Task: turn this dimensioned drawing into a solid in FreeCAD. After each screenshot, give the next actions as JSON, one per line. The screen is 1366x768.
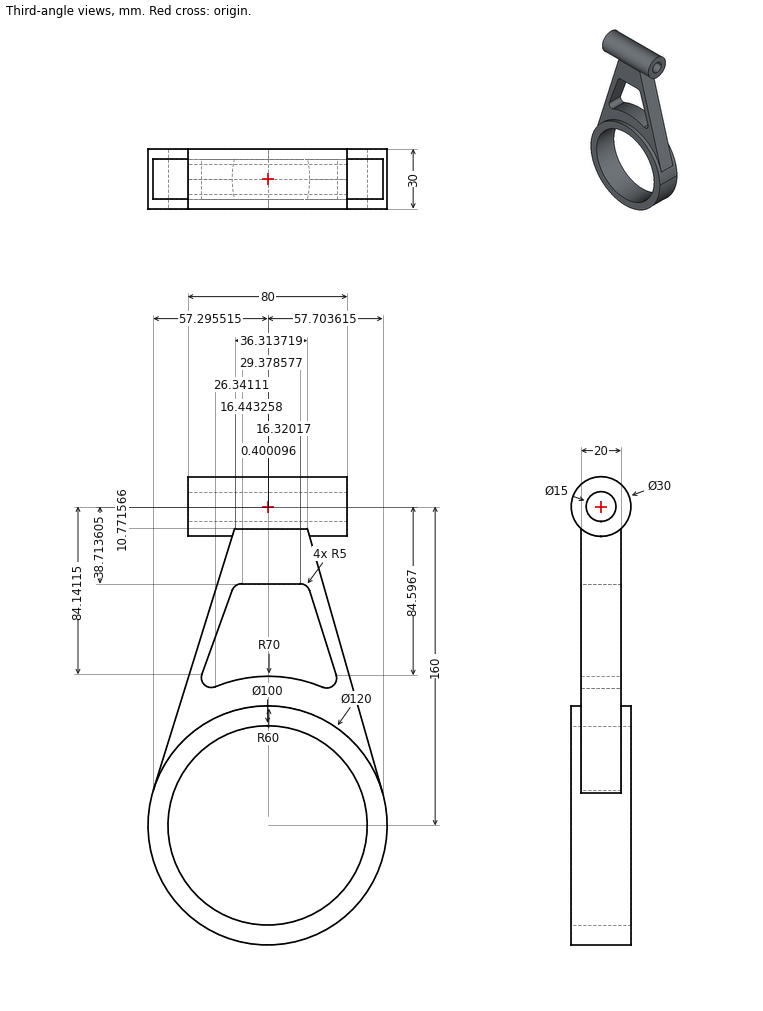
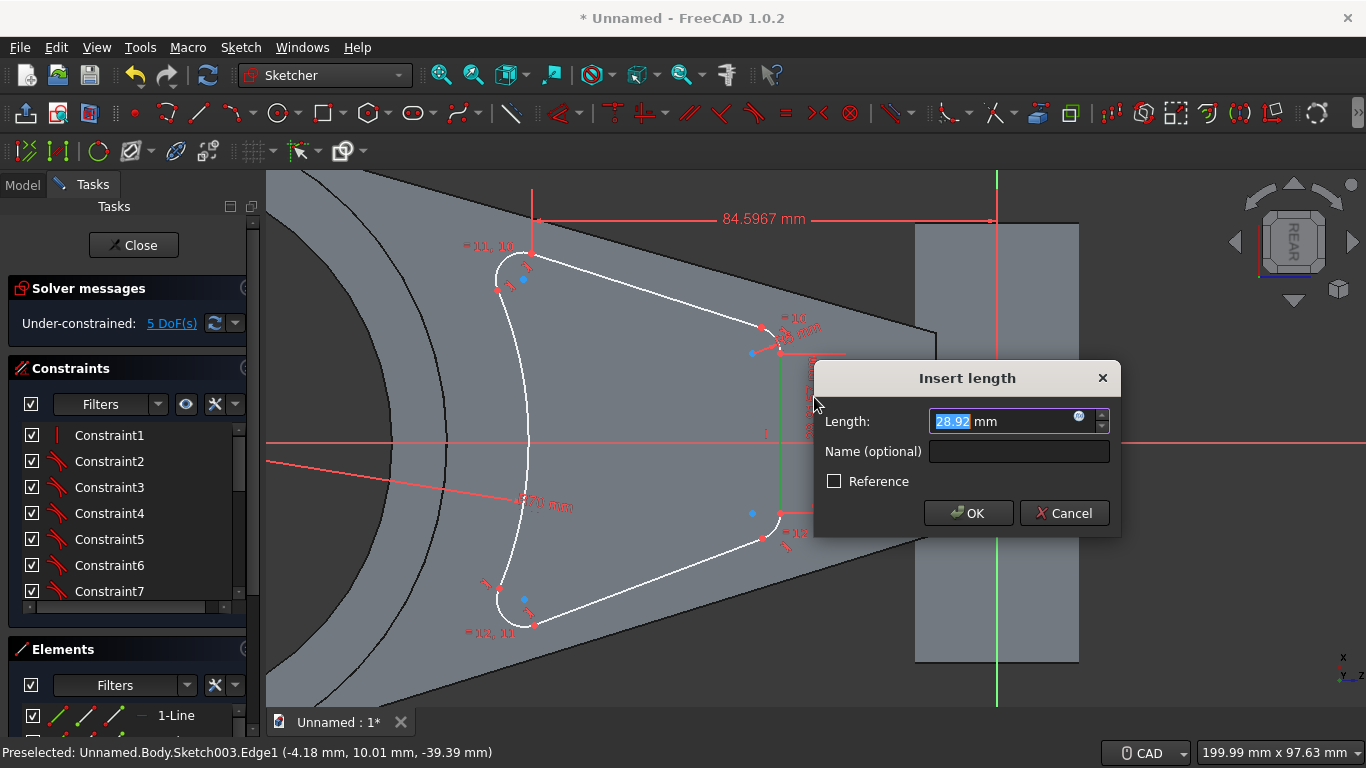
{"action": "type", "text": "29.378577"}
{"action": "key", "text": "Return"}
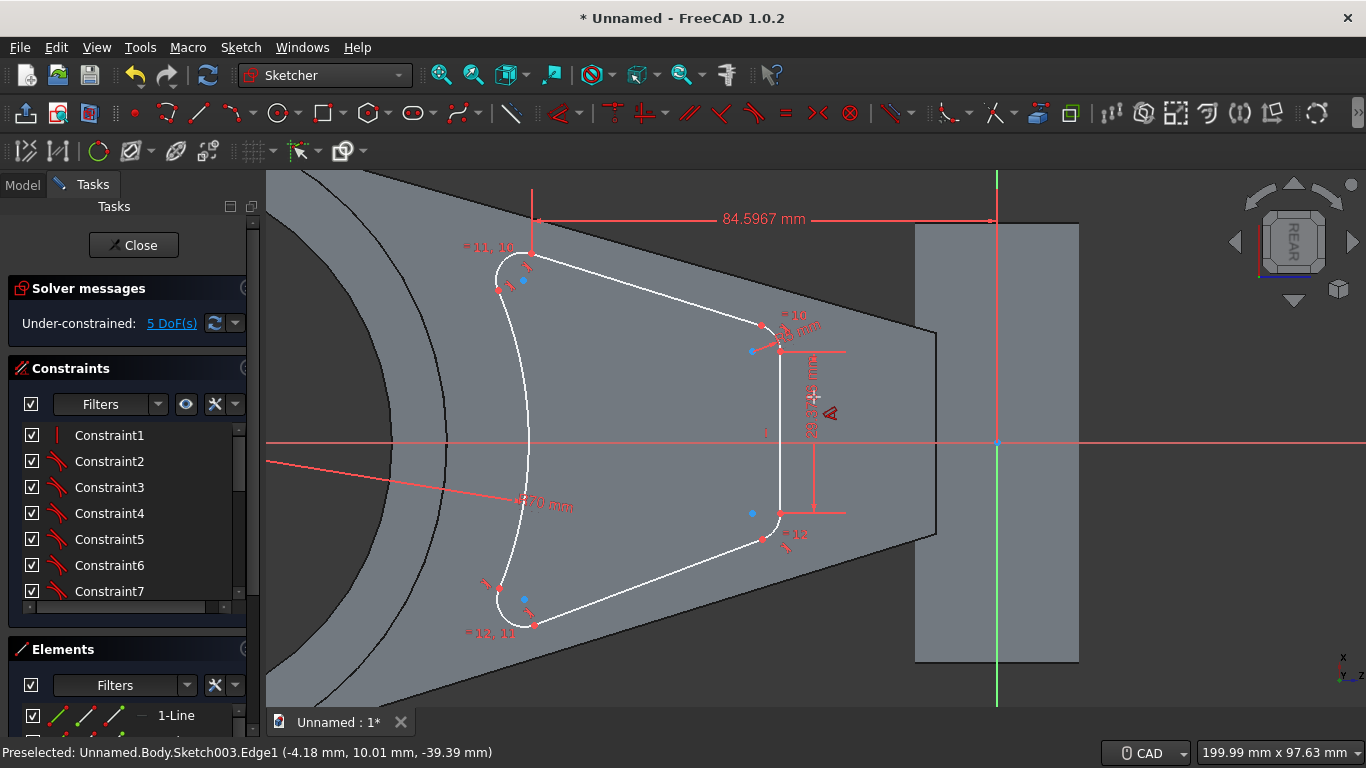
{"action": "left_click", "coordinate": [780, 352]}
{"action": "left_click", "coordinate": [1031, 397]}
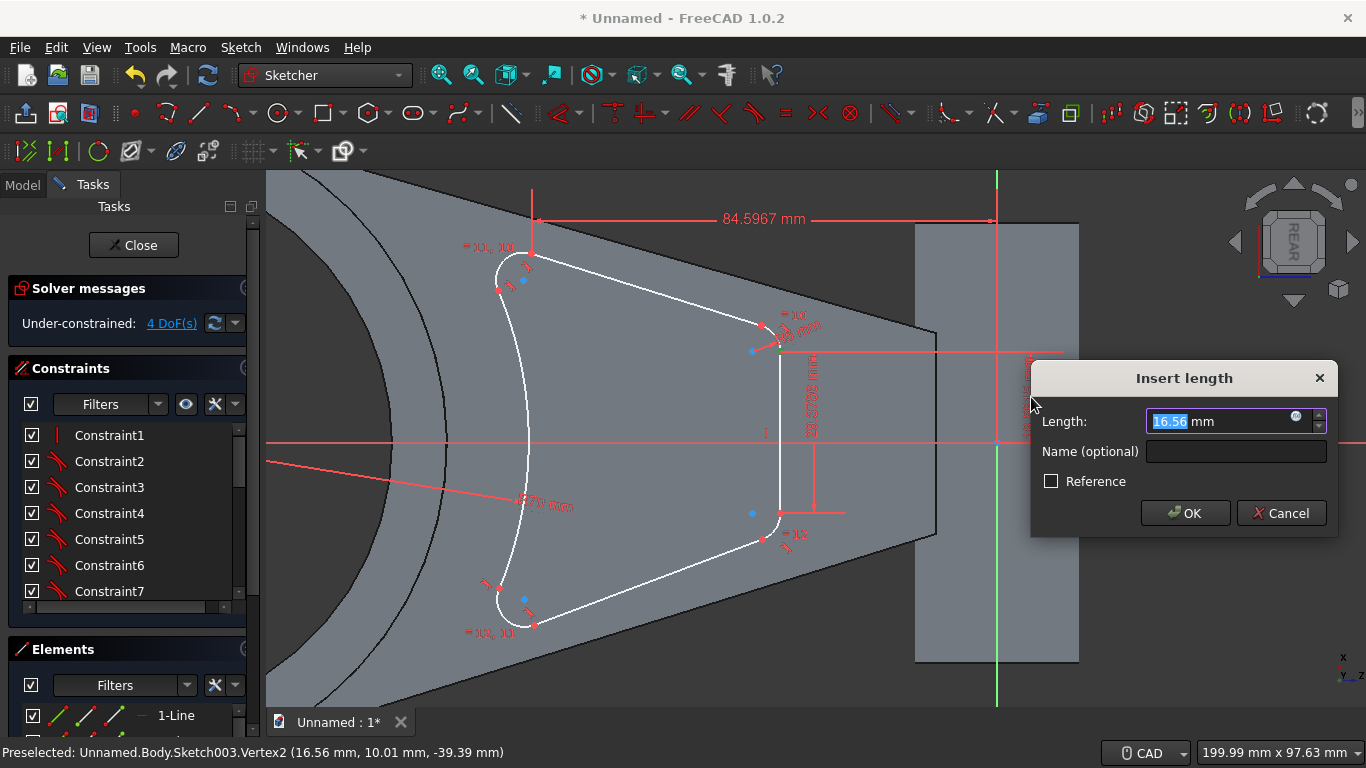
{"action": "type", "text": "16.32017"}
{"action": "key", "text": "Return"}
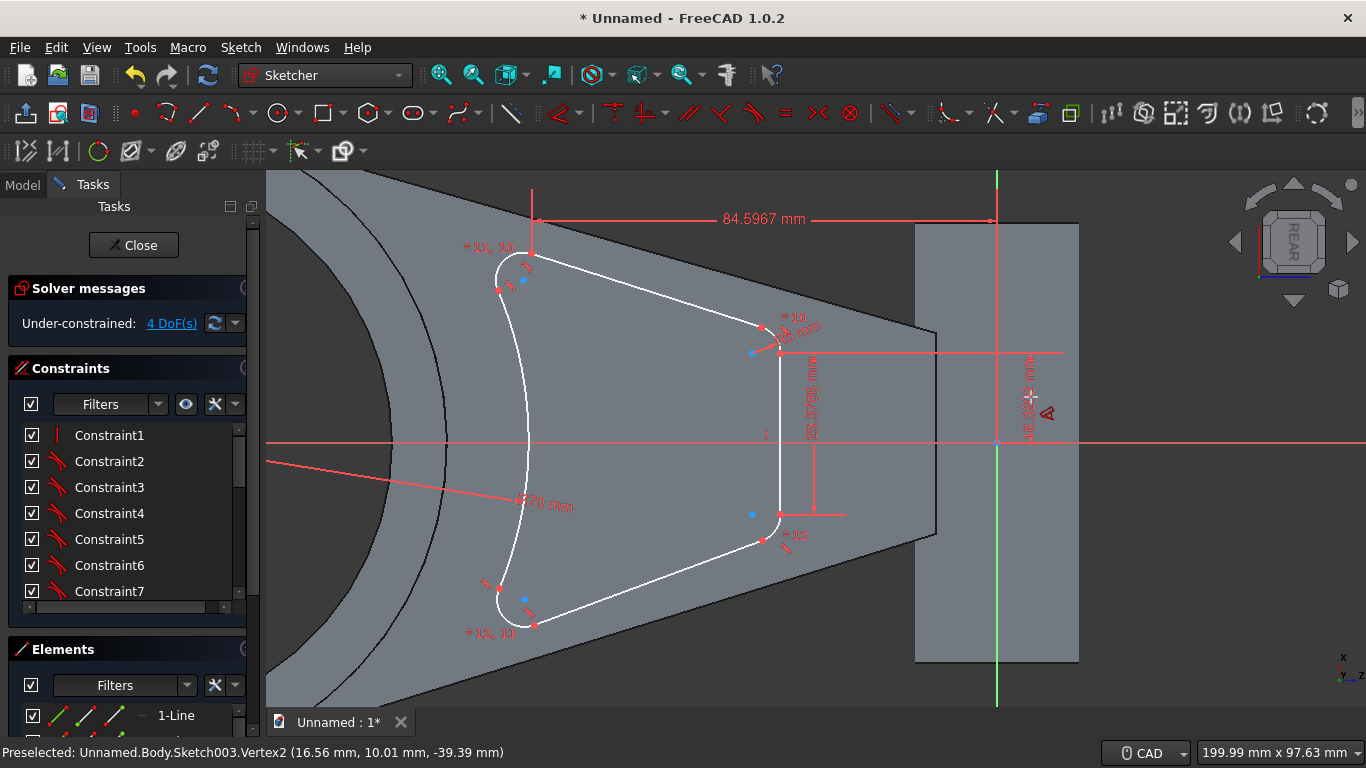
{"action": "left_click", "coordinate": [534, 625]}
{"action": "left_click", "coordinate": [766, 659]}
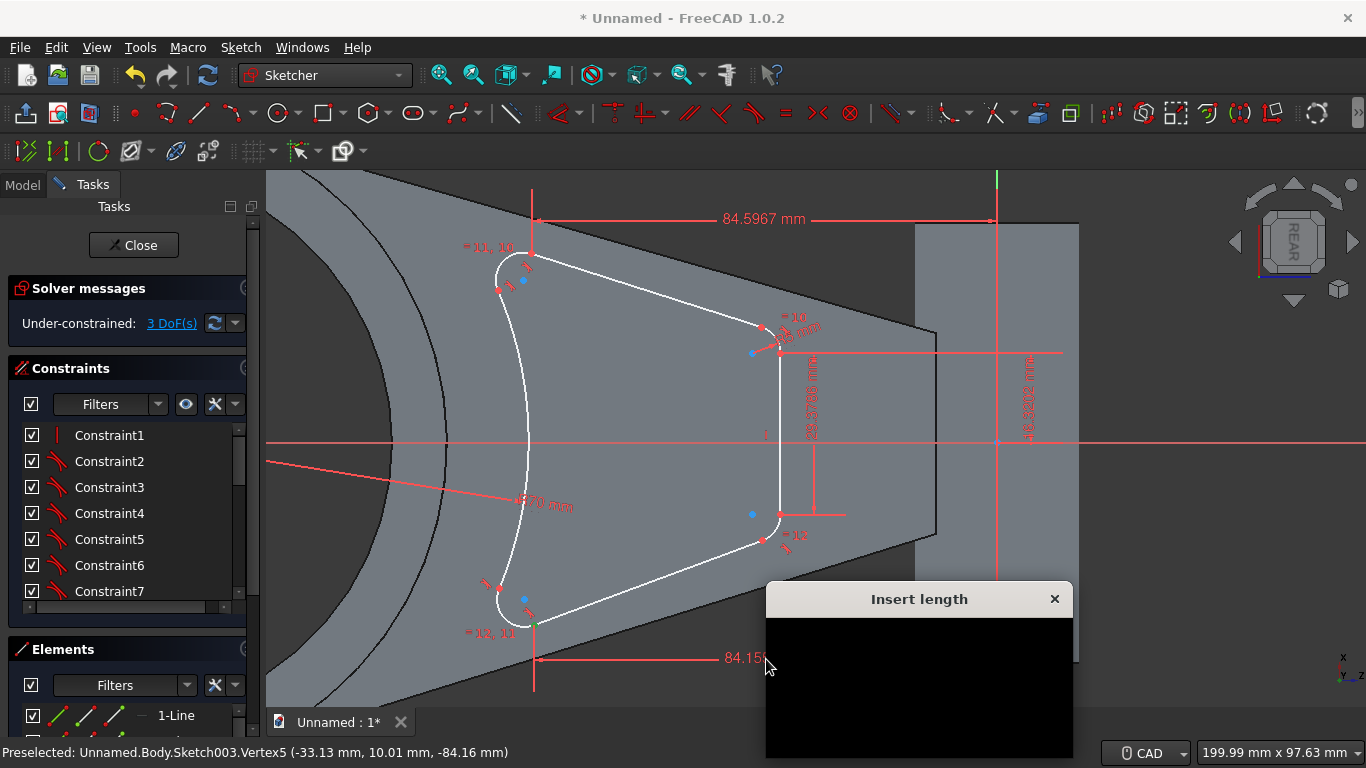
{"action": "type", "text": "84.14115"}
{"action": "key", "text": "Return"}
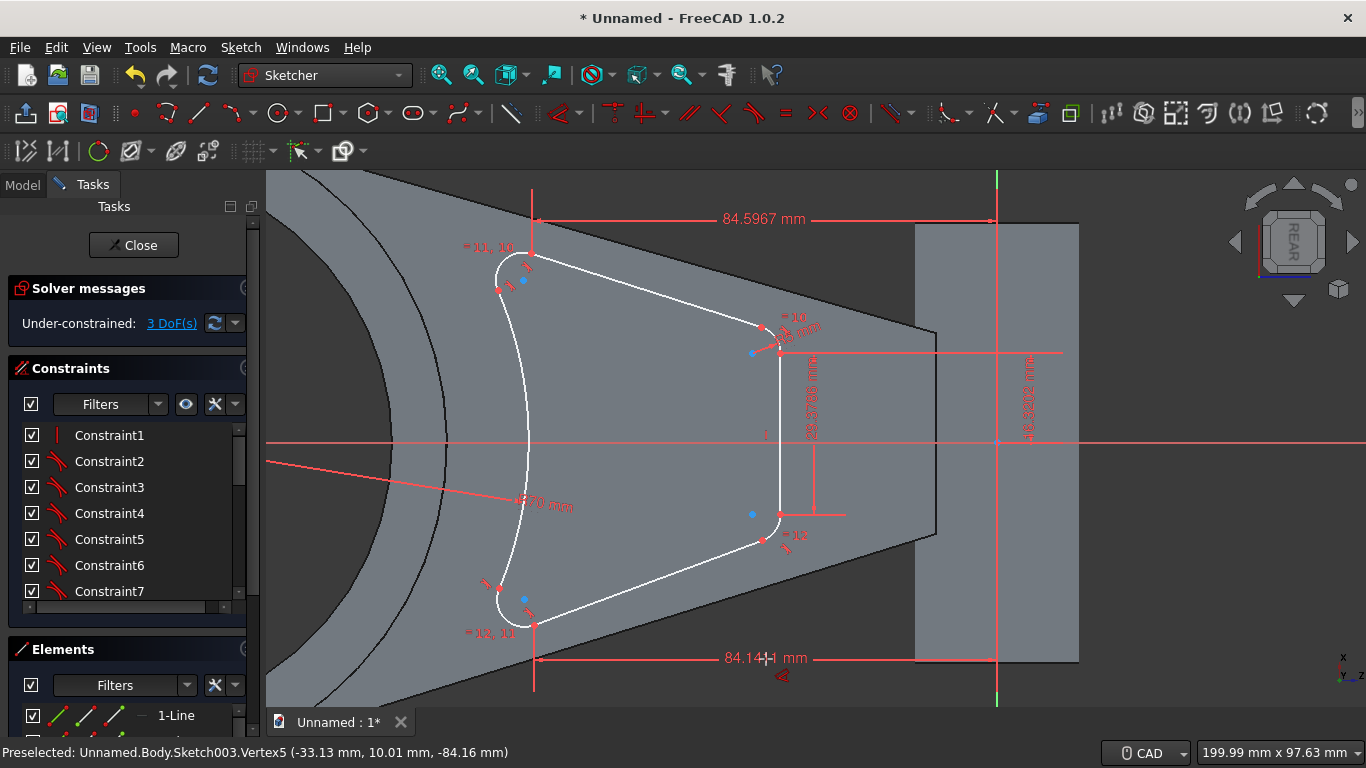
{"action": "left_click", "coordinate": [499, 589]}
{"action": "left_click", "coordinate": [1031, 516]}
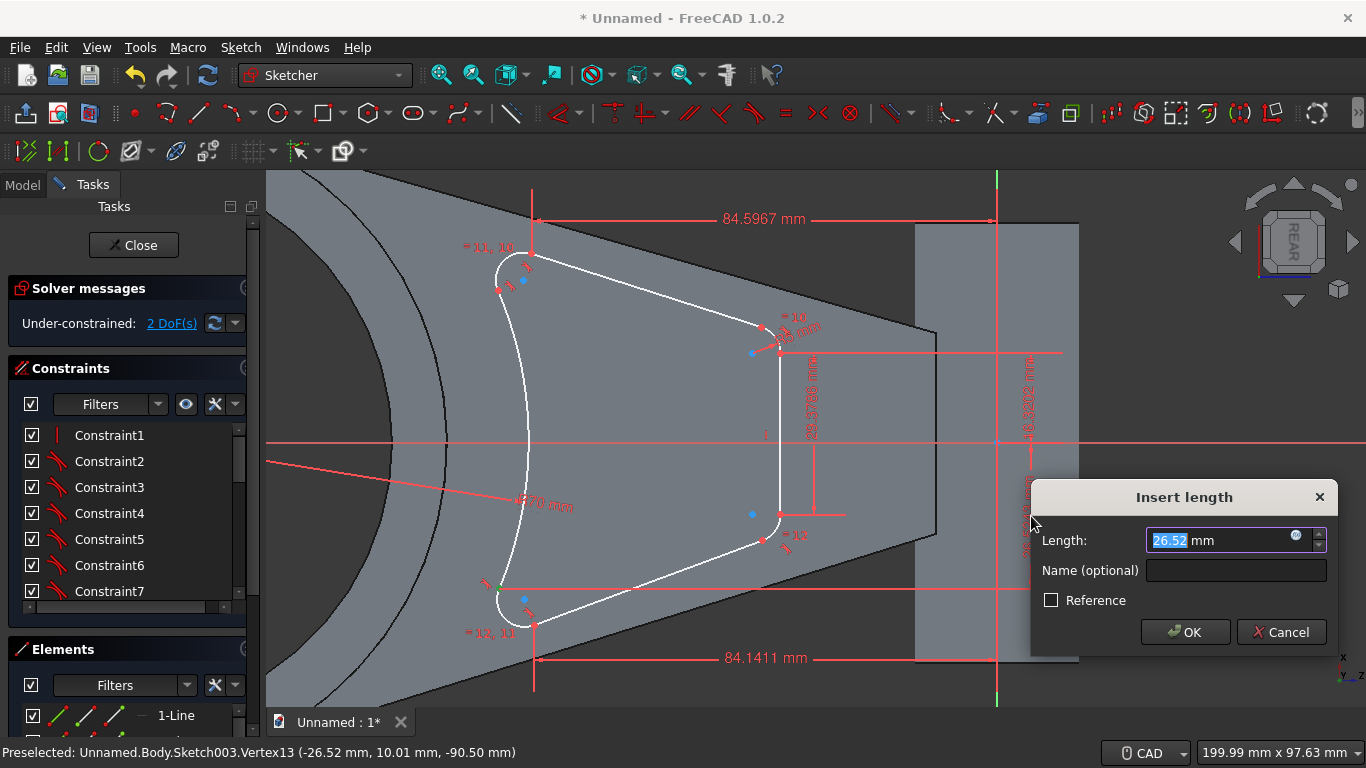
{"action": "type", "text": "26.34111"}
{"action": "key", "text": "Return"}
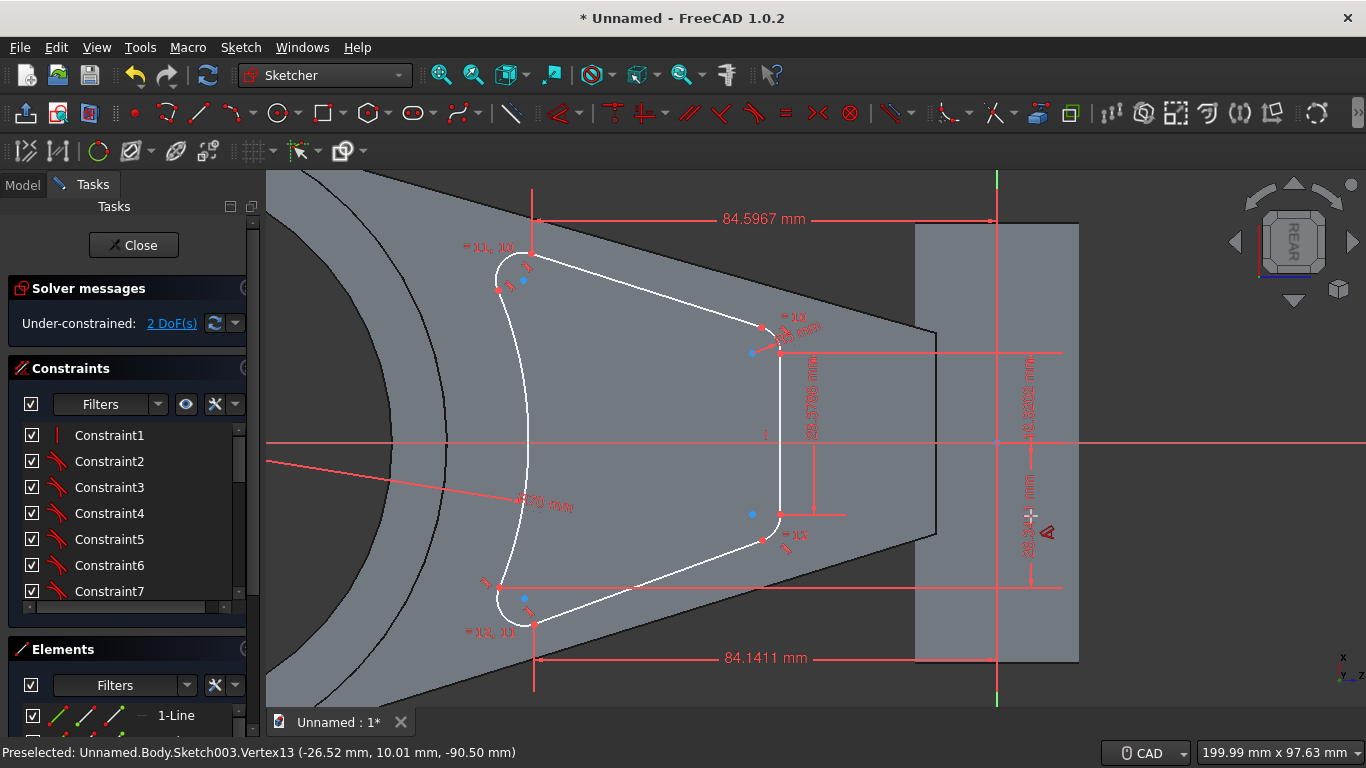
{"action": "scroll", "coordinate": [1201, 437], "scroll_direction": "down", "scroll_amount": 1}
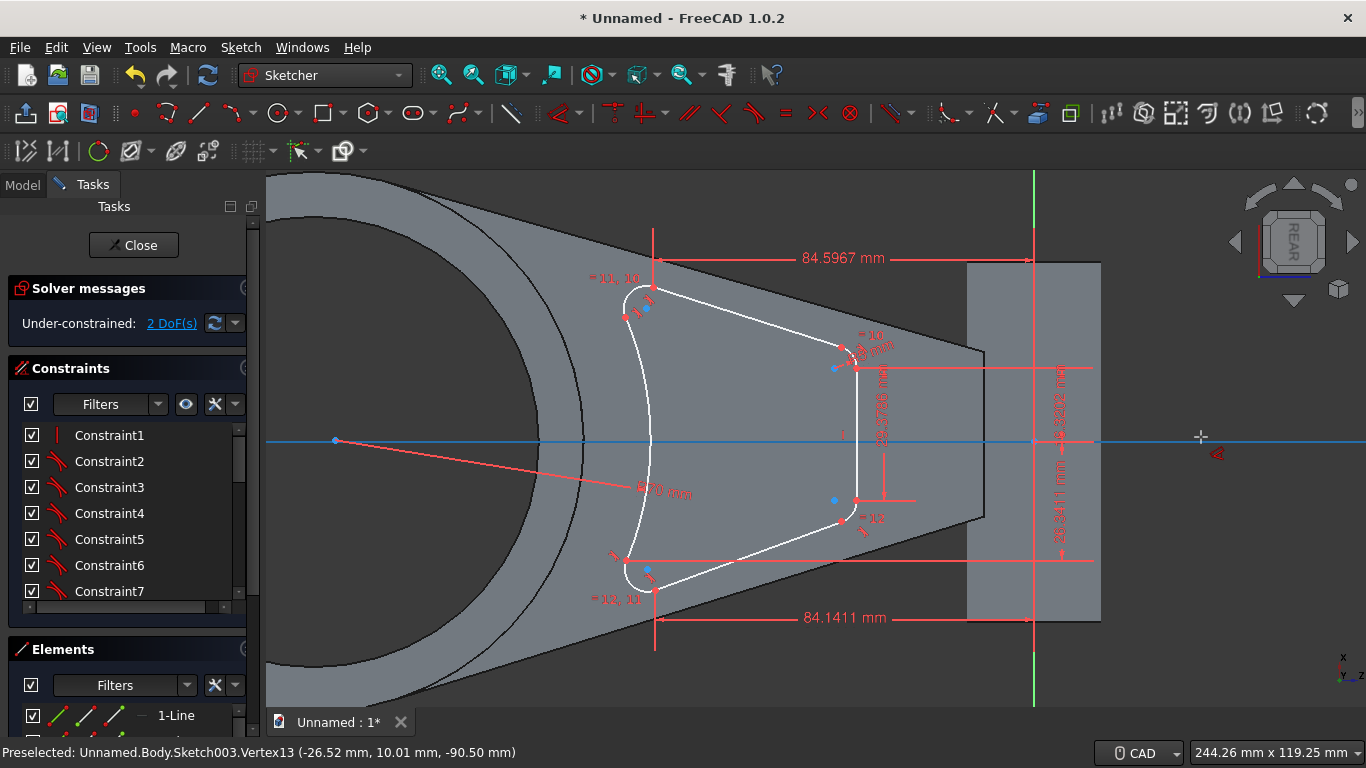
{"action": "scroll", "coordinate": [335, 440], "scroll_direction": "up", "scroll_amount": 16}